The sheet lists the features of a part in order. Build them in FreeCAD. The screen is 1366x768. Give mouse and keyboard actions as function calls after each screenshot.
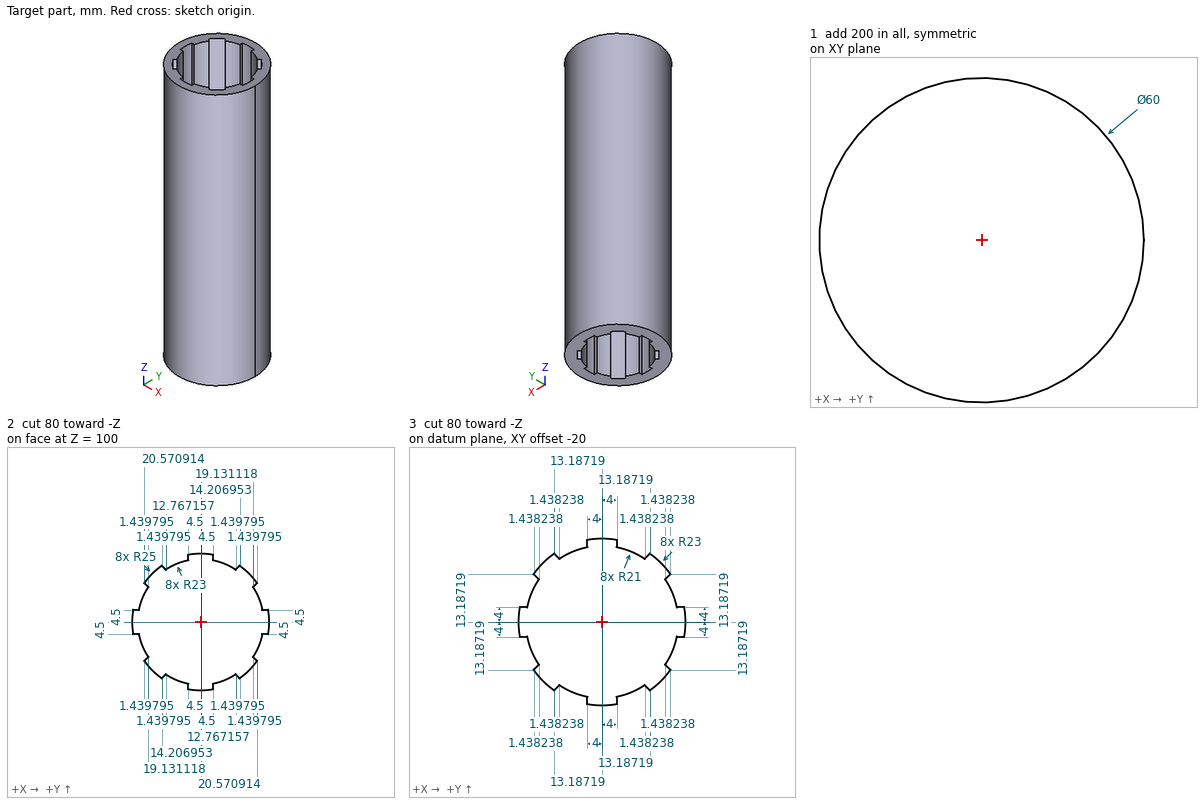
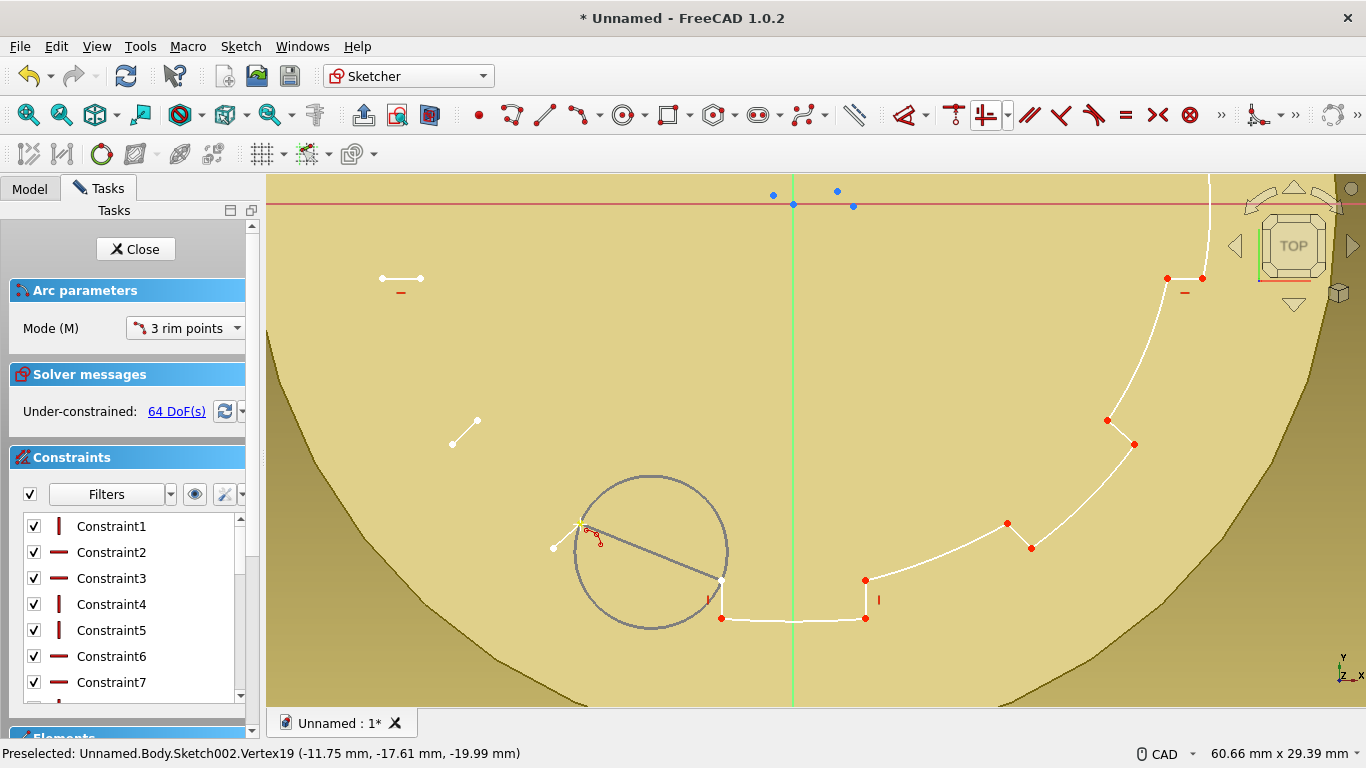
scroll(648, 556, up, 4)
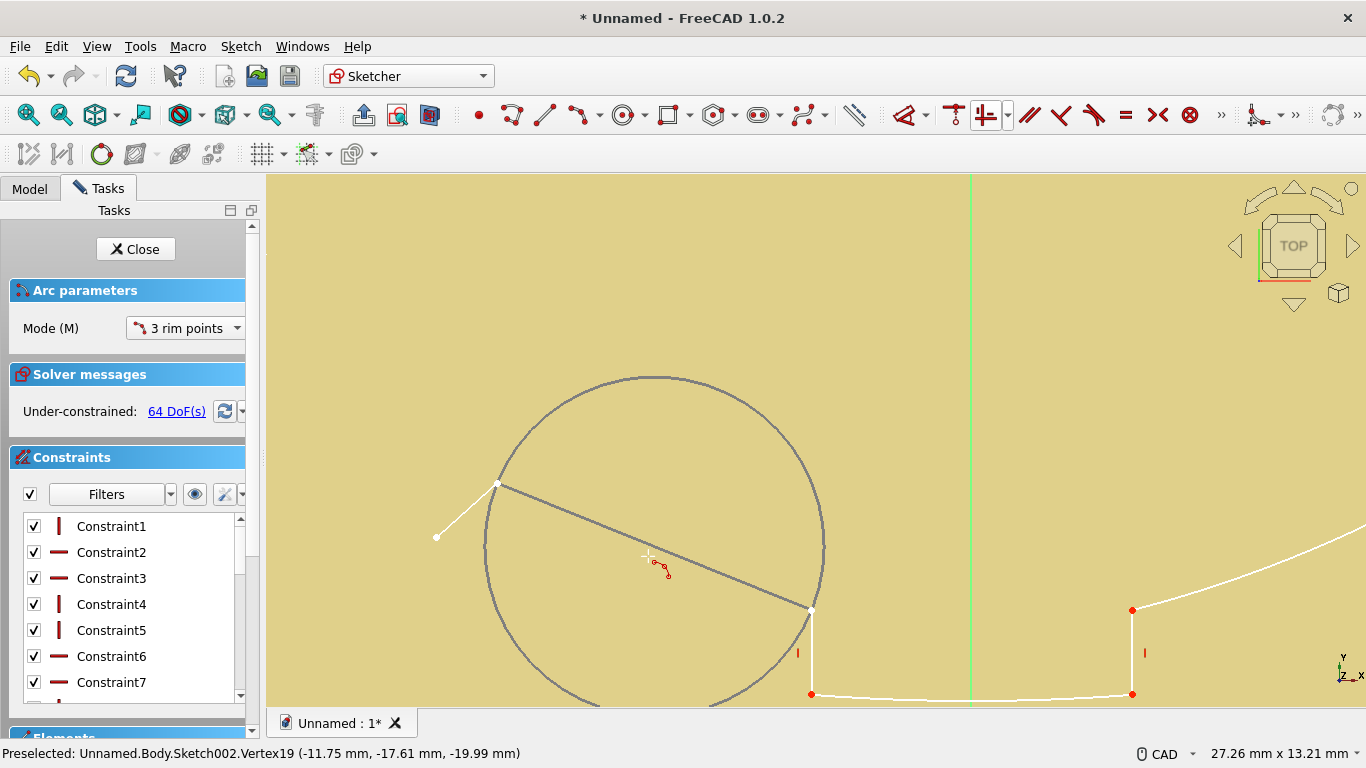
click(647, 555)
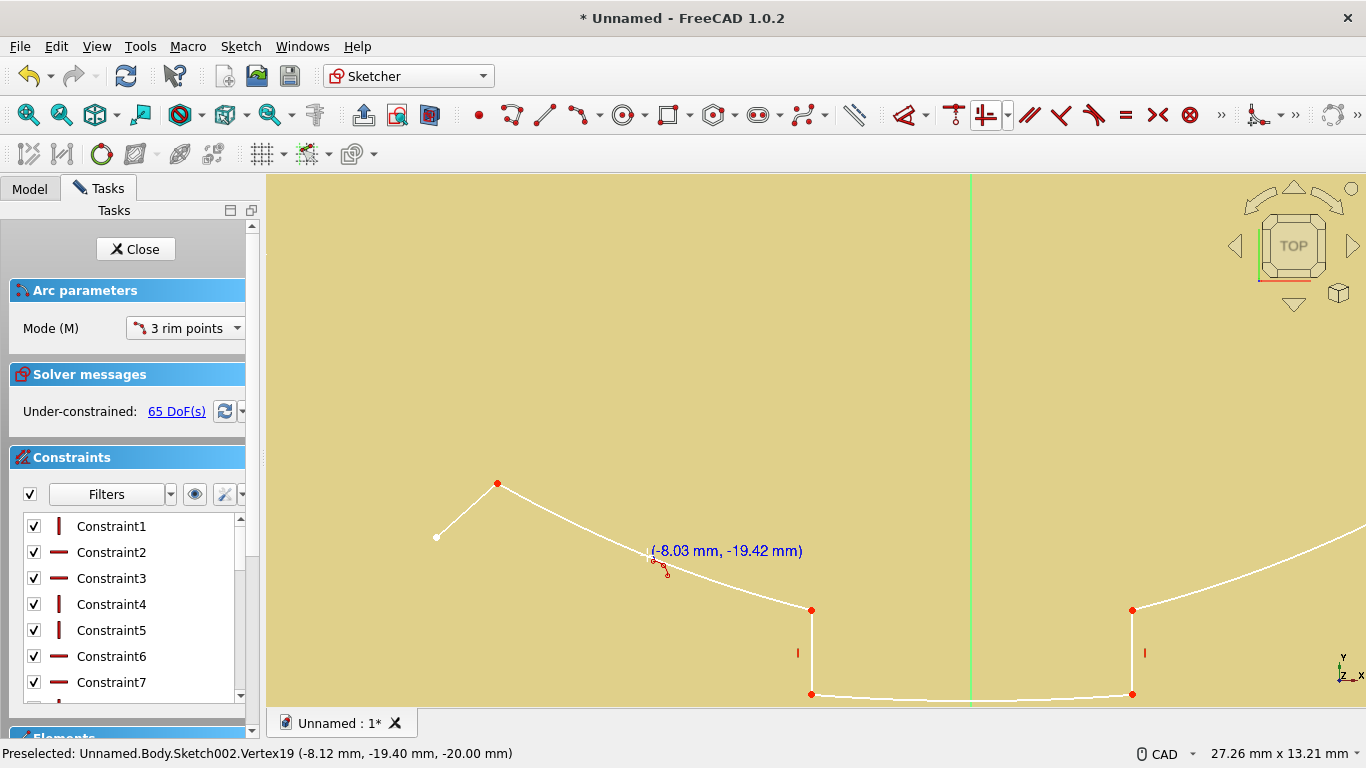
click(437, 538)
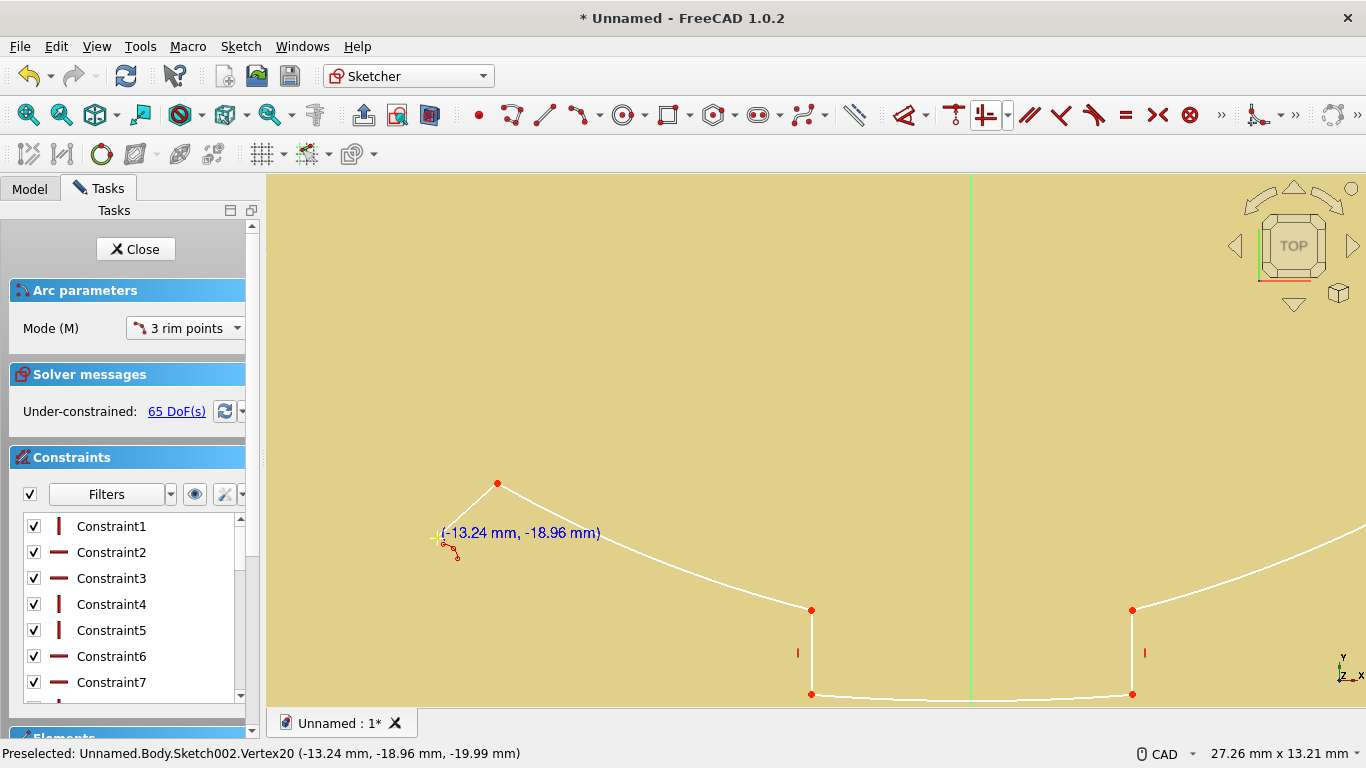
scroll(703, 573, down, 9)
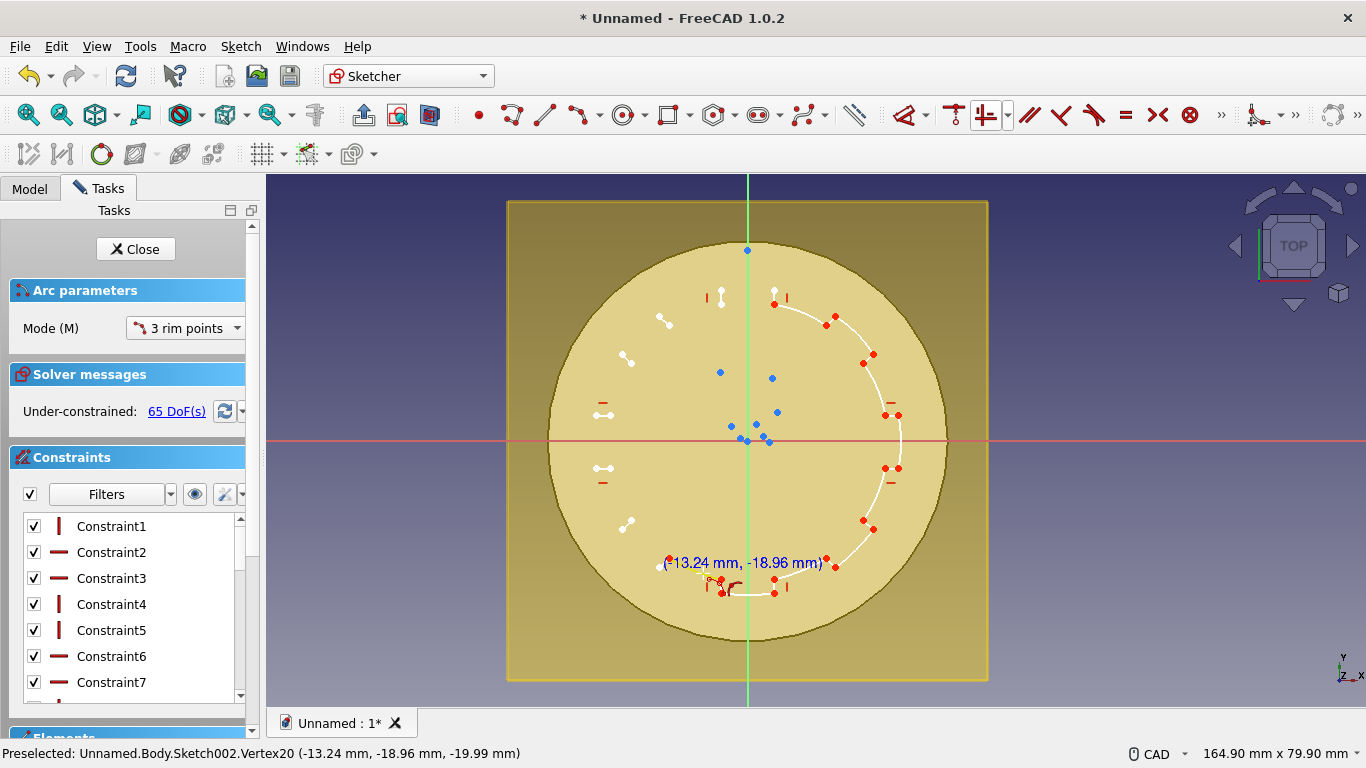
scroll(622, 529, up, 5)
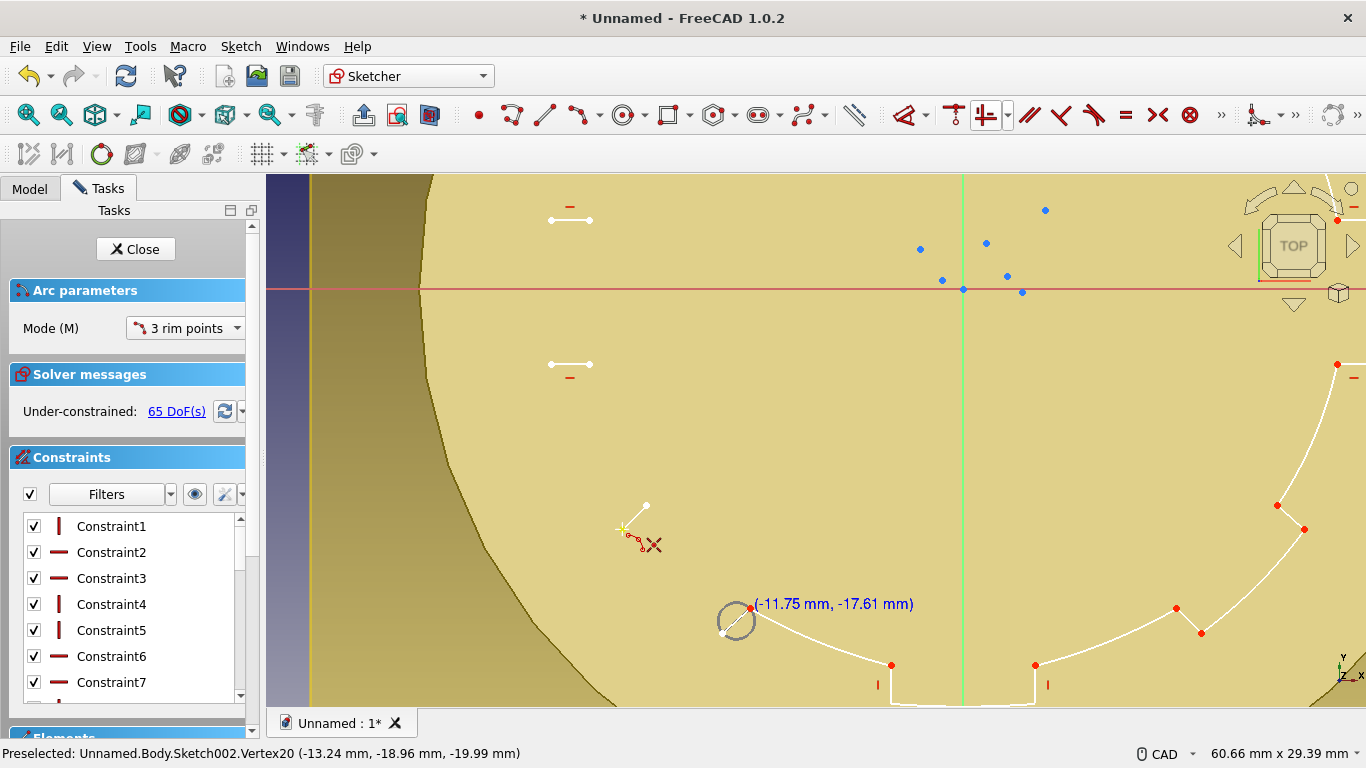
click(622, 530)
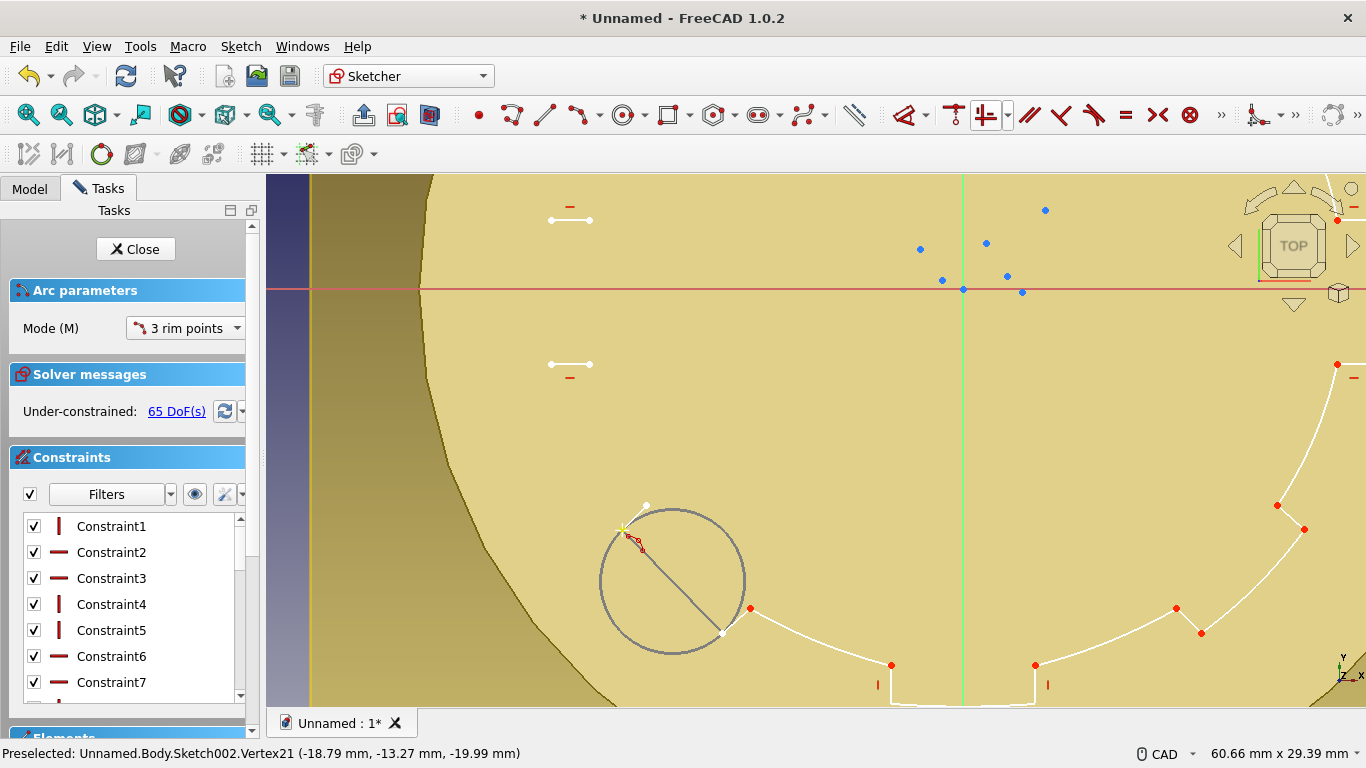
scroll(668, 584, up, 5)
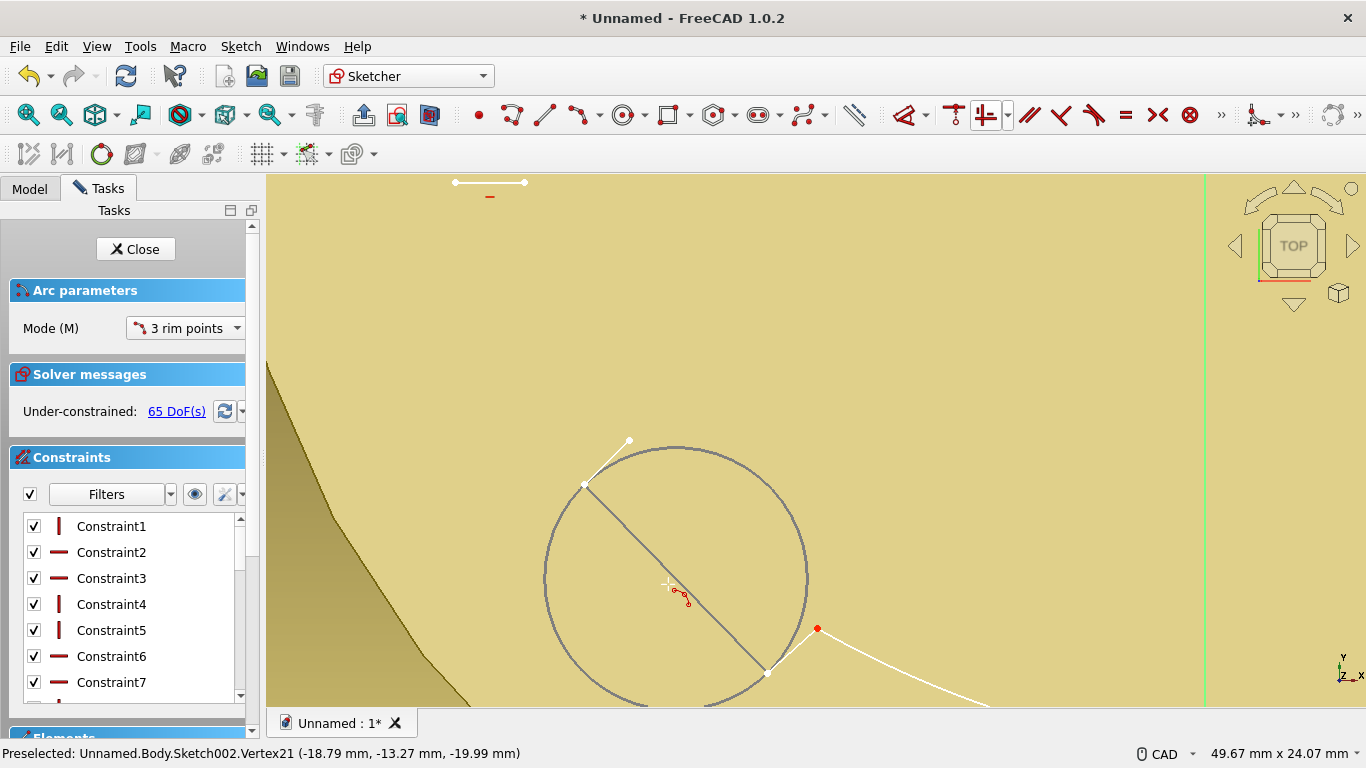
click(668, 583)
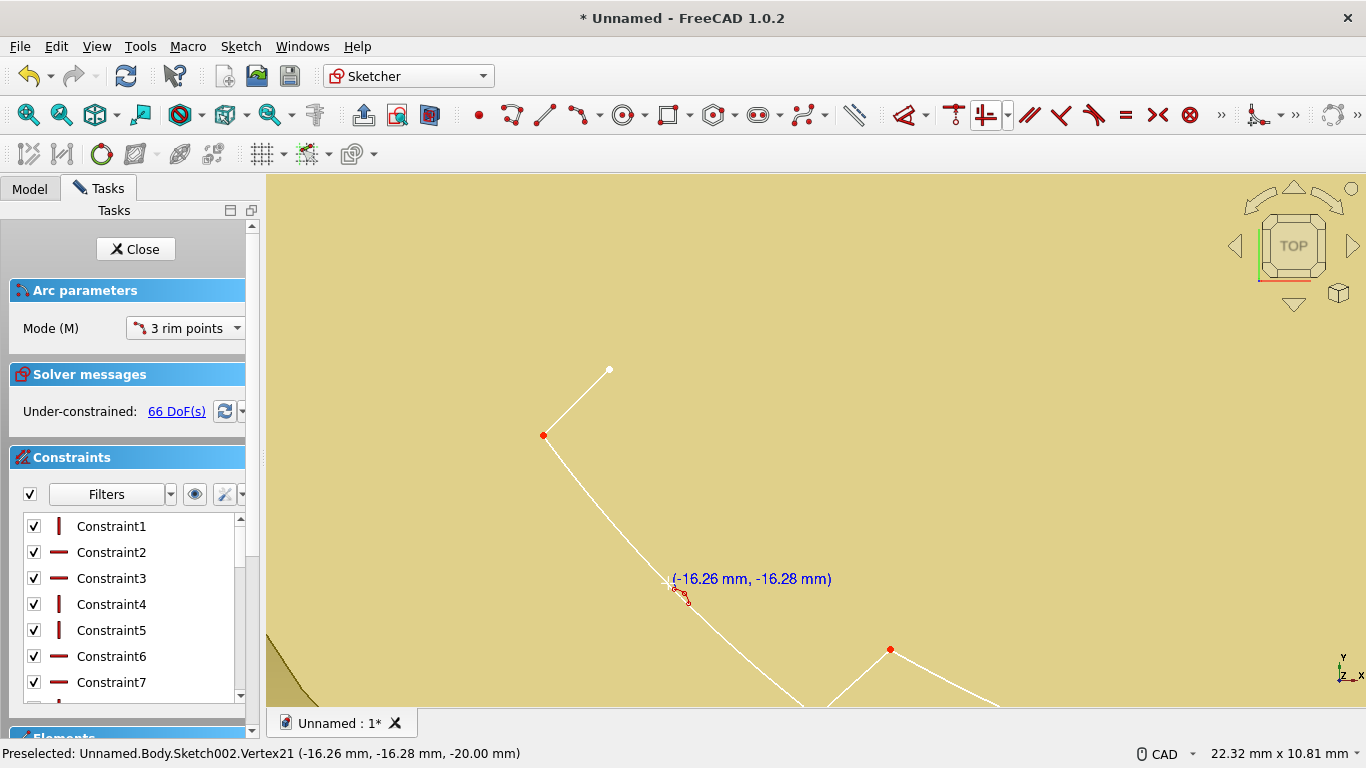
scroll(635, 544, down, 10)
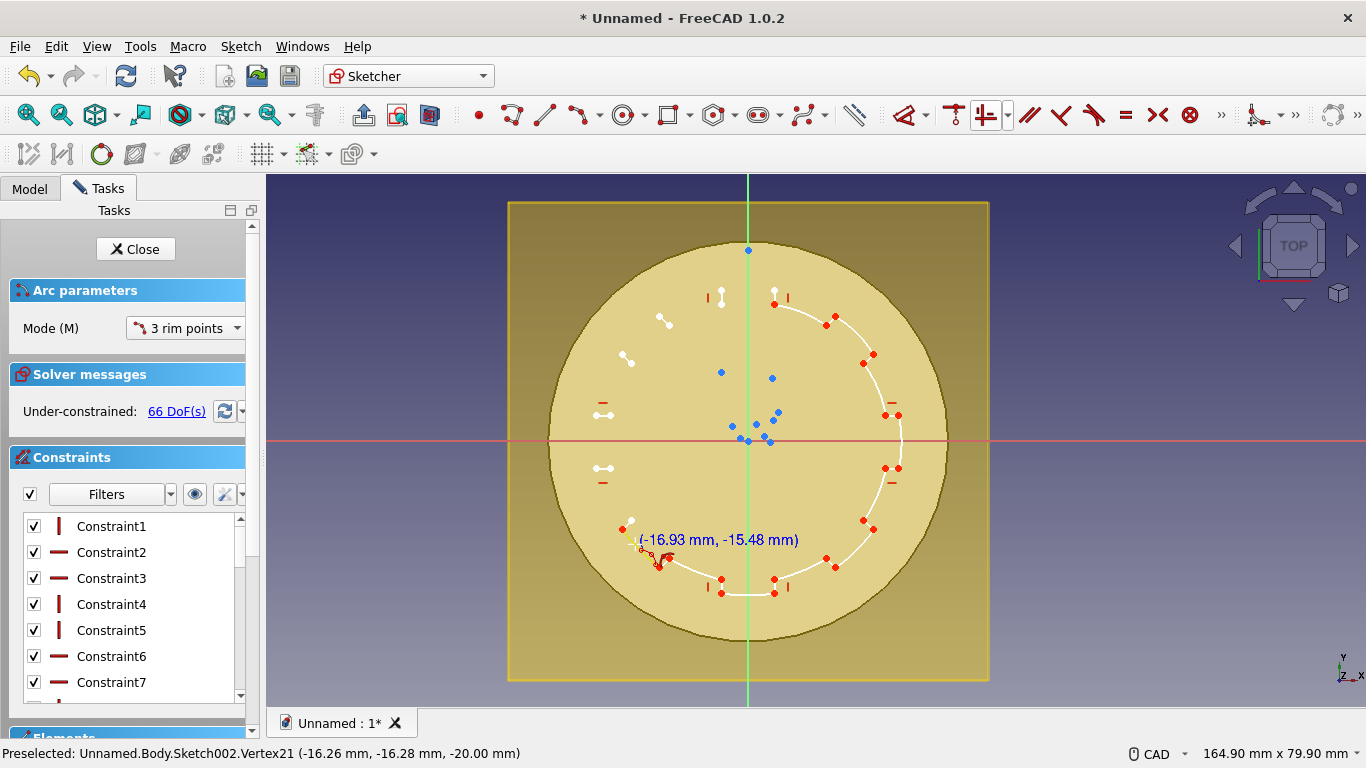
scroll(632, 520, up, 5)